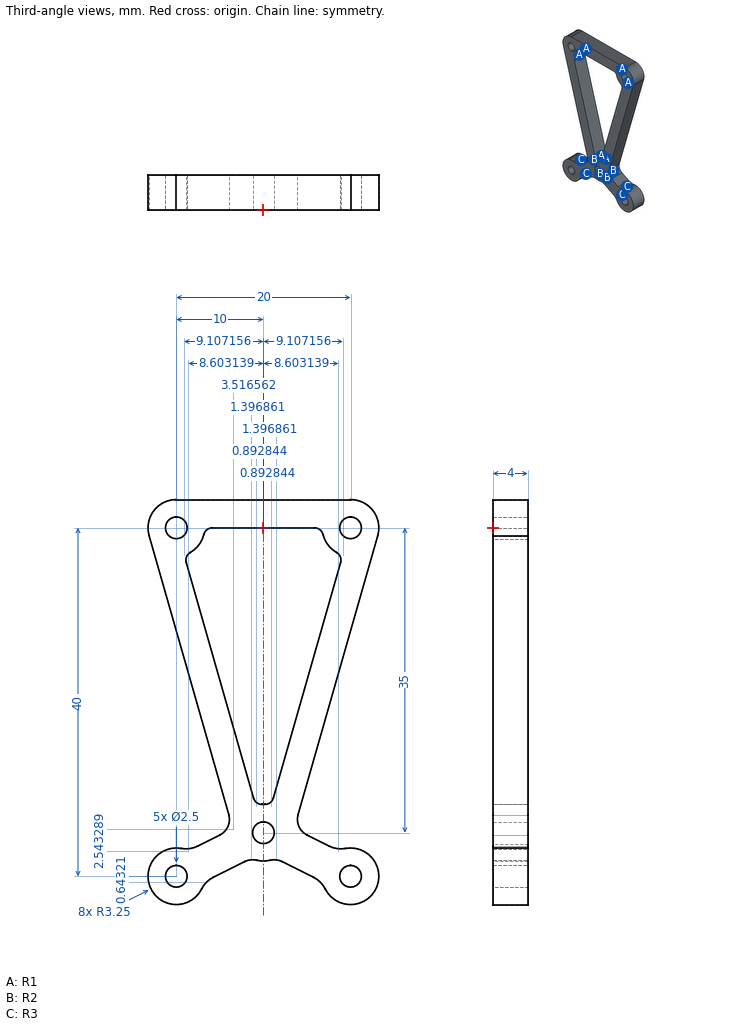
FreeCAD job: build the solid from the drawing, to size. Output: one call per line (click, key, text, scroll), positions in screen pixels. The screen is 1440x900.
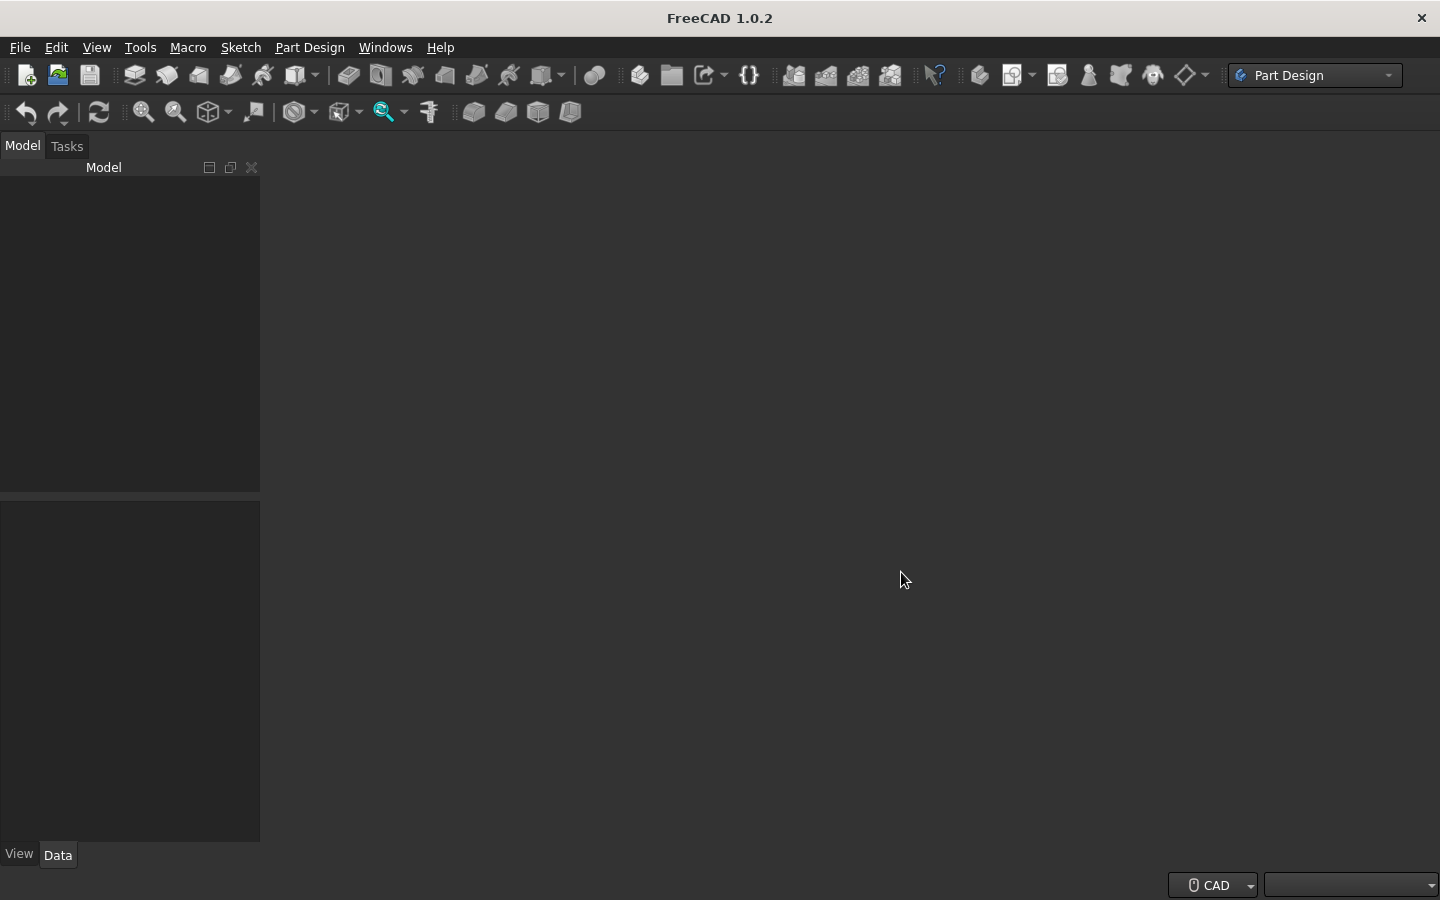
key(ctrl+n)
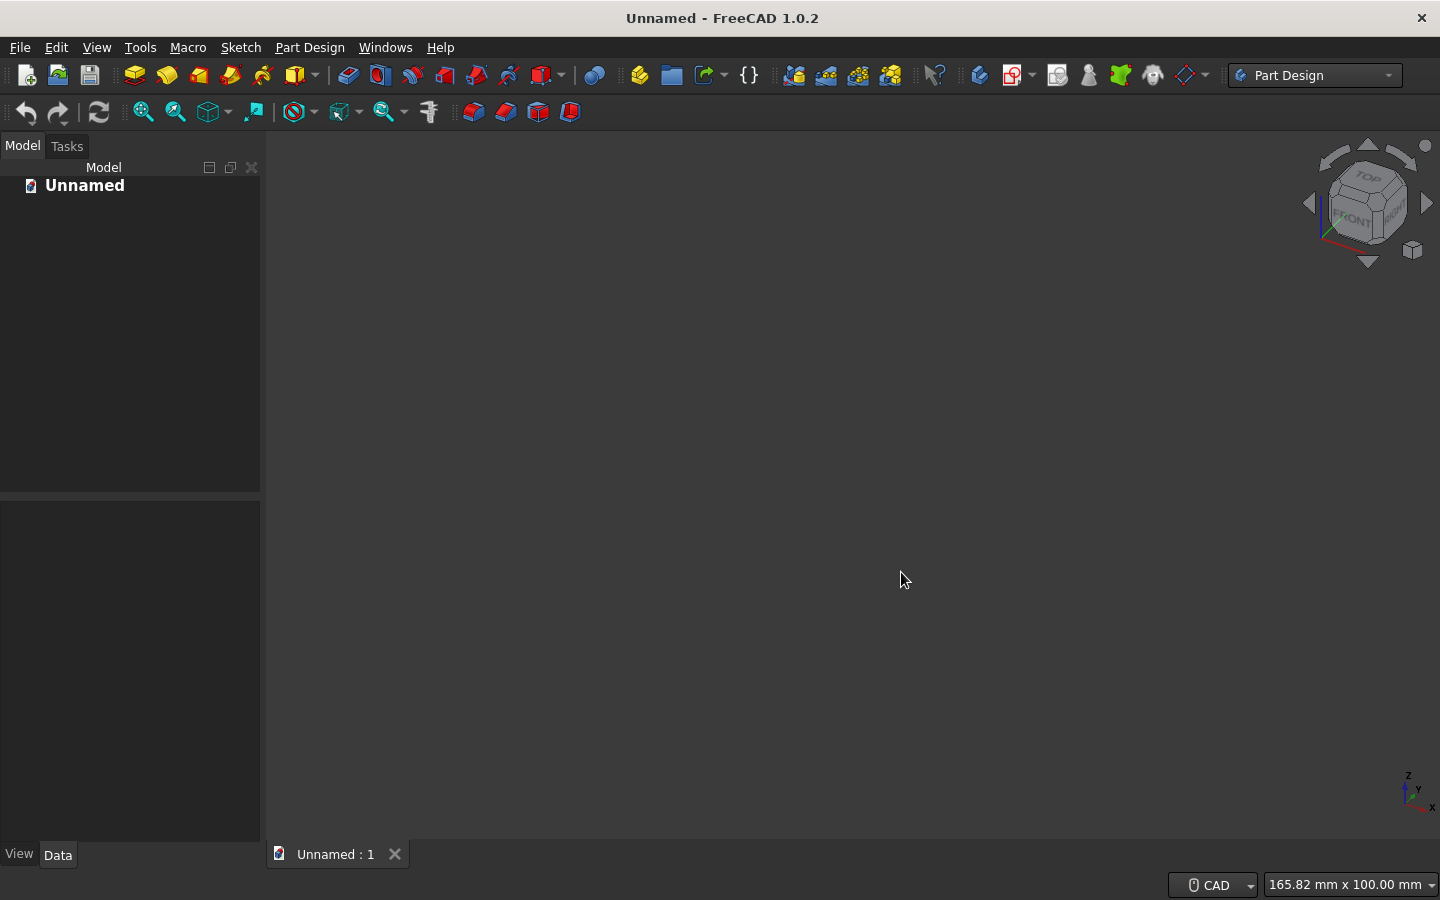
click(1012, 76)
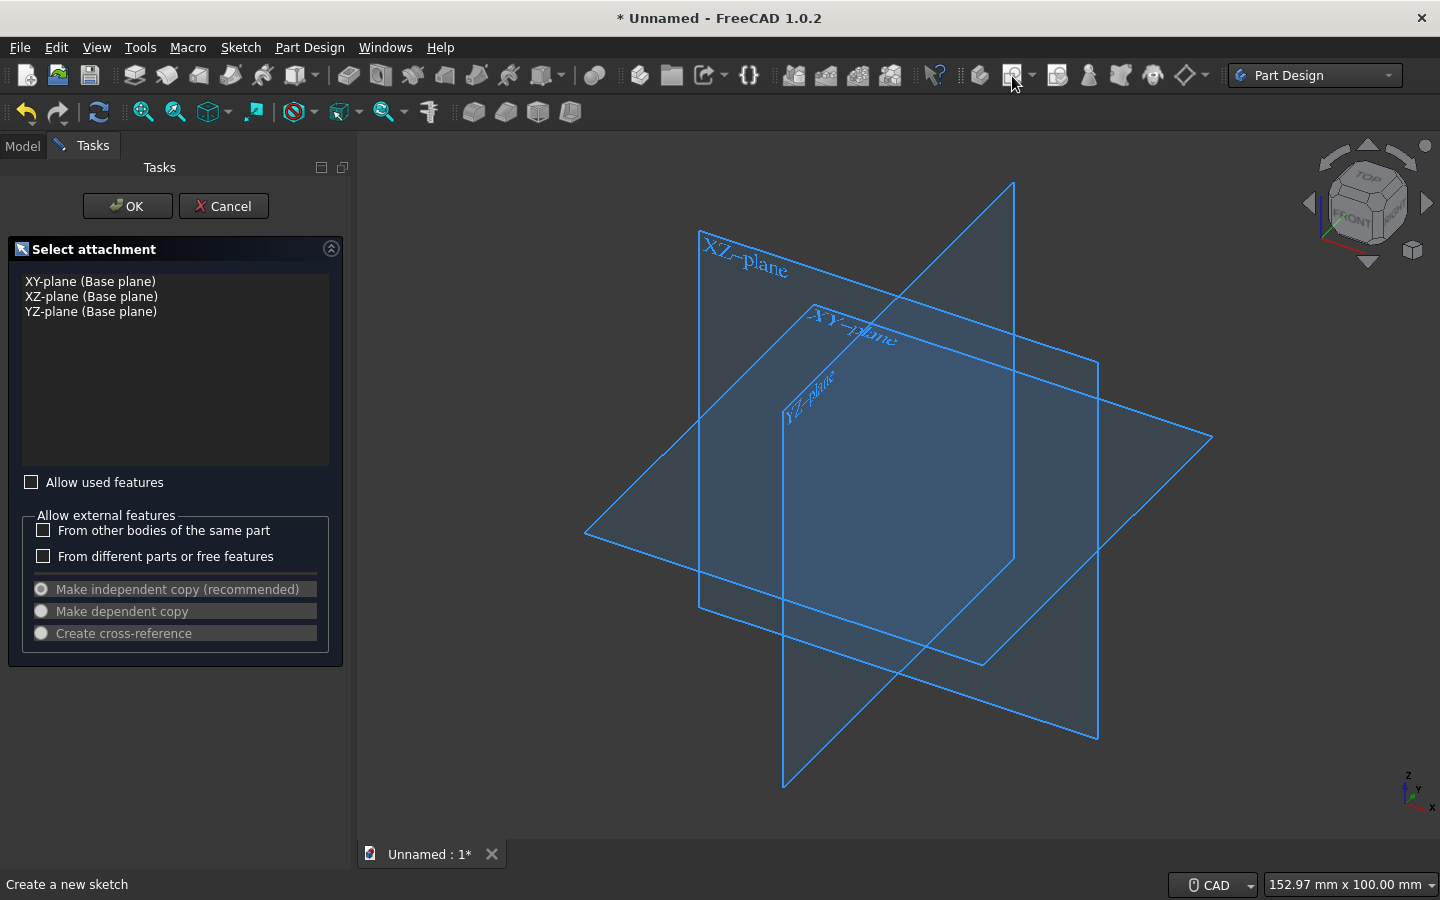
click(82, 296)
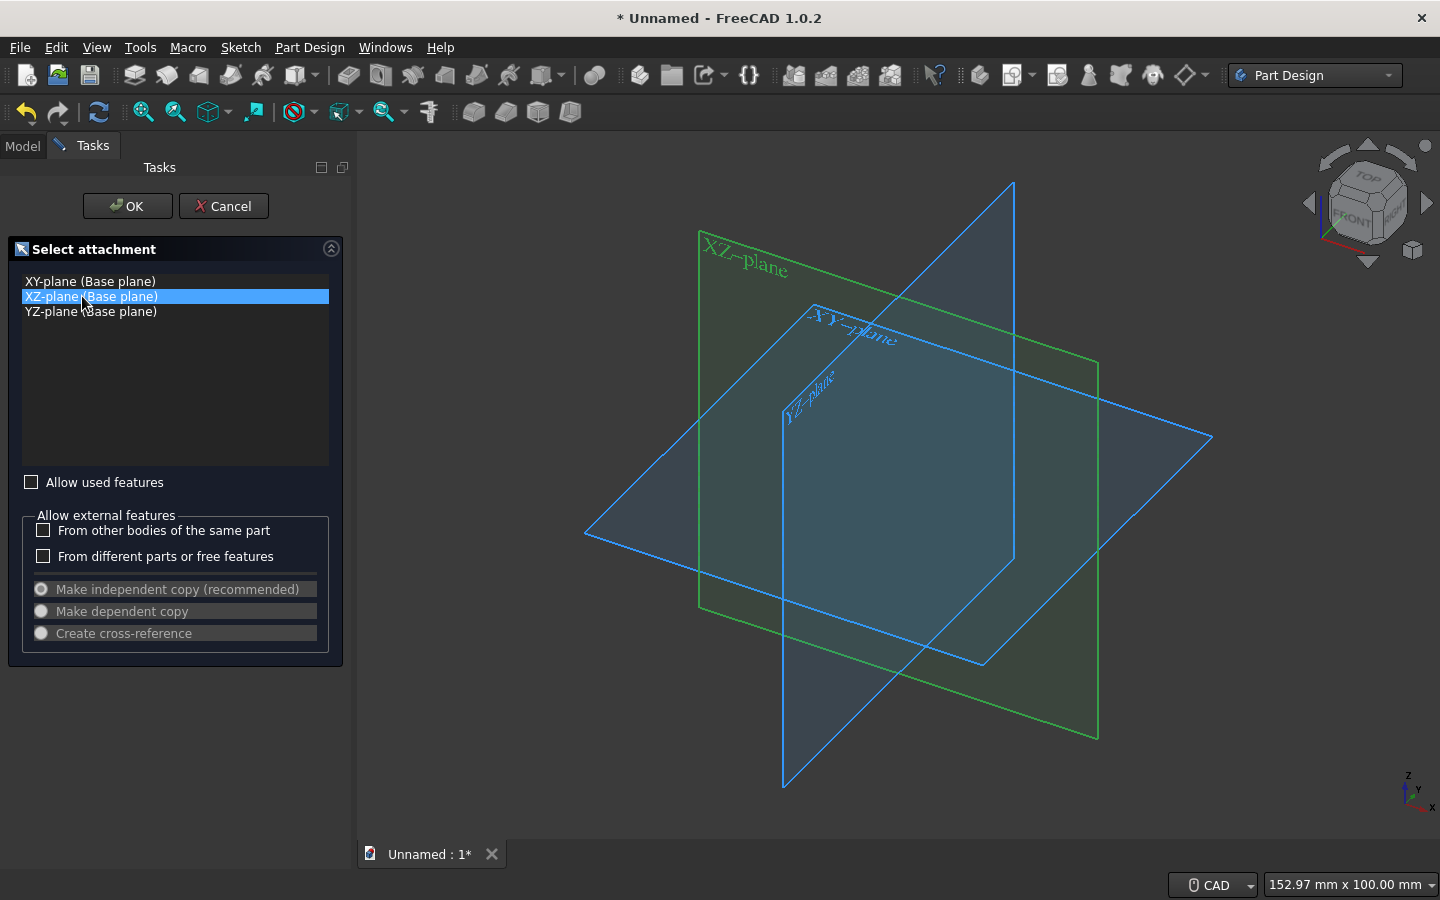
click(128, 206)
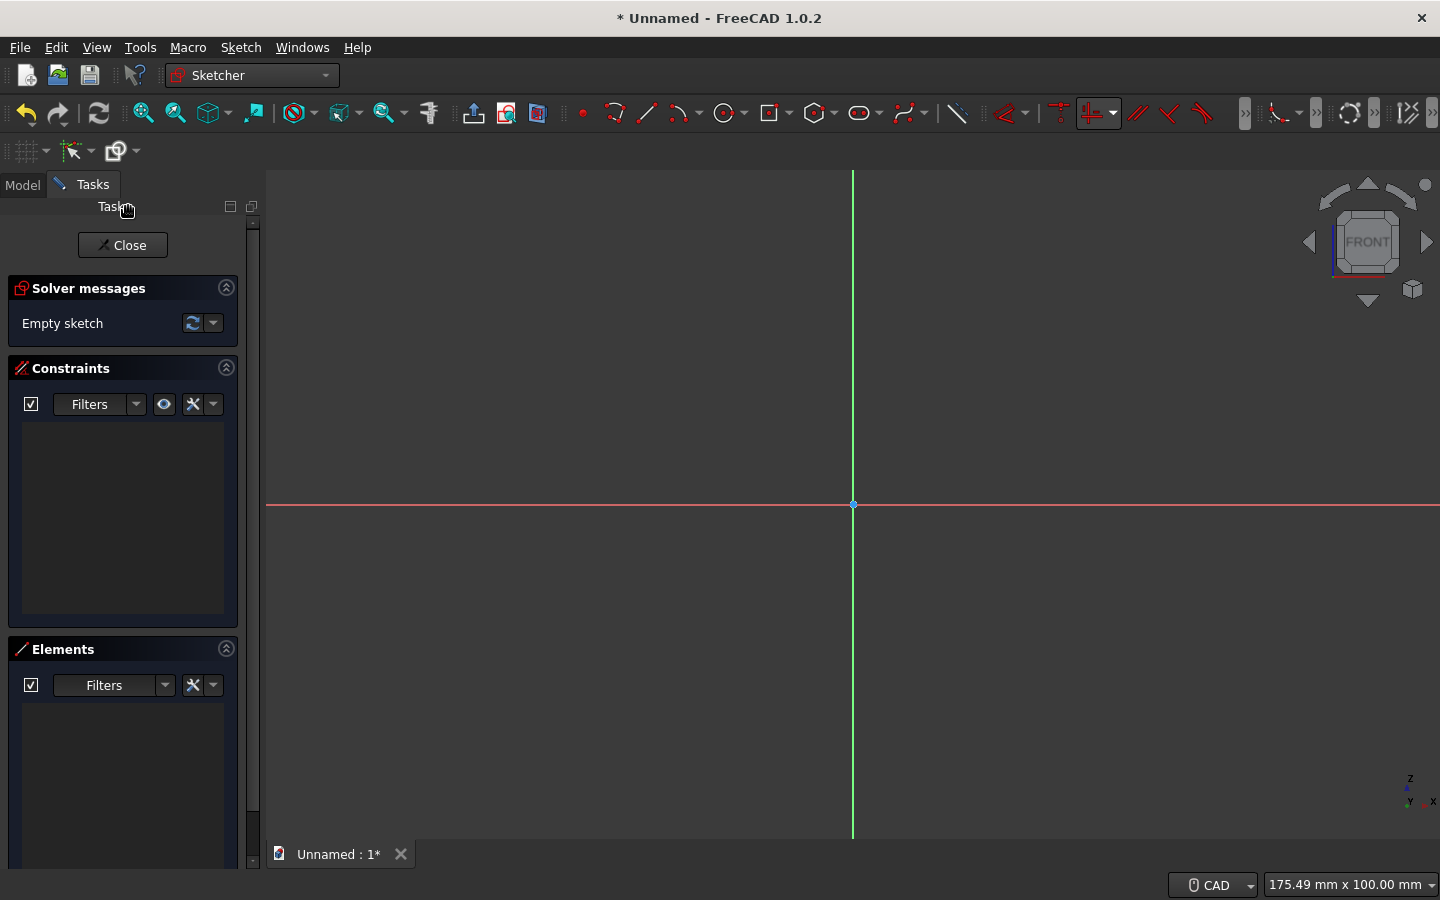
scroll(992, 811, up, 2)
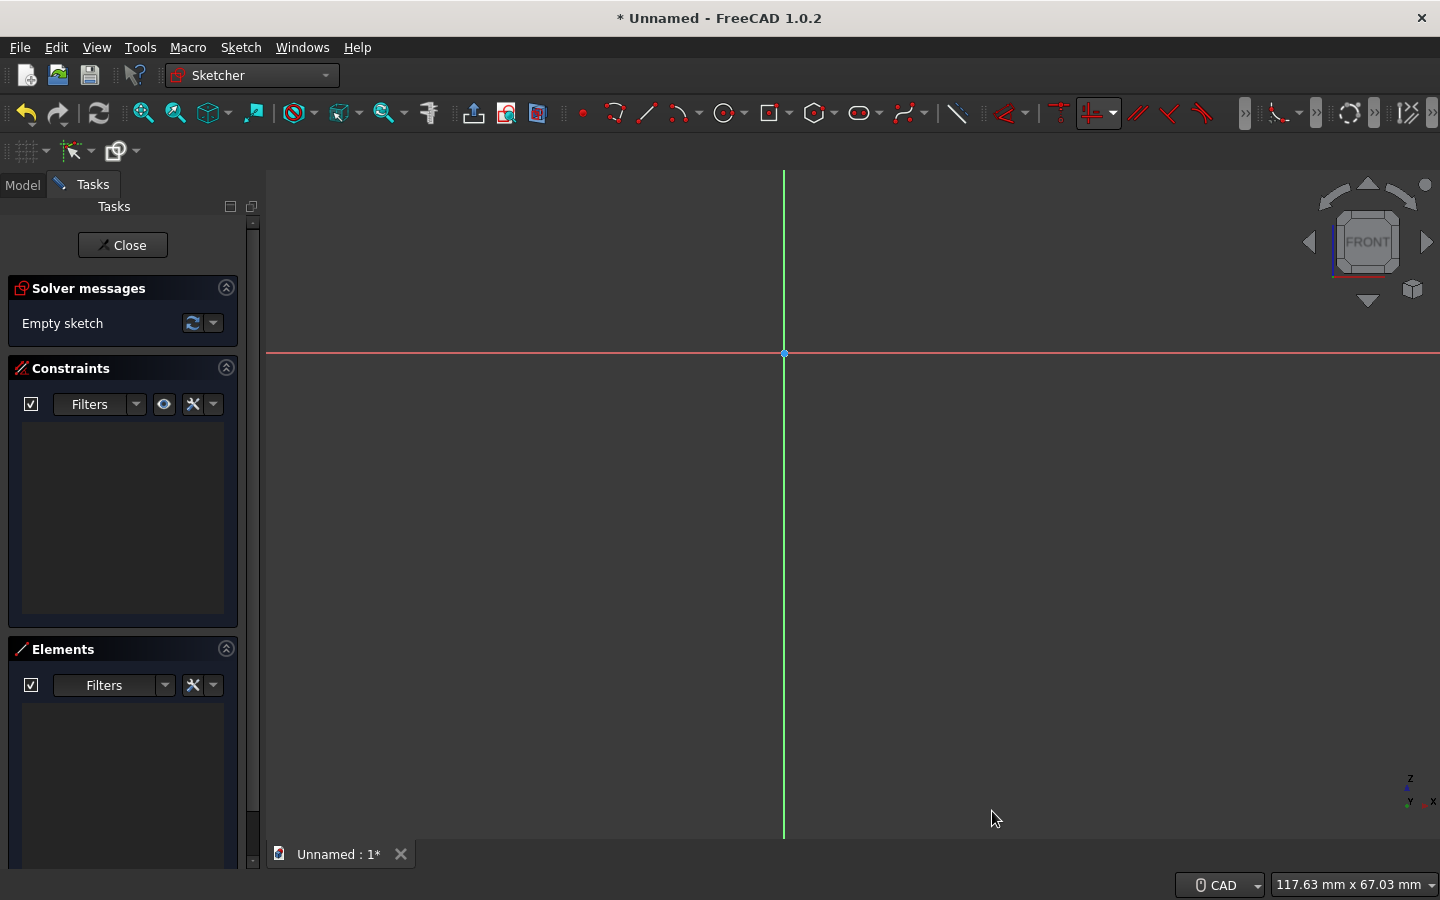
click(616, 114)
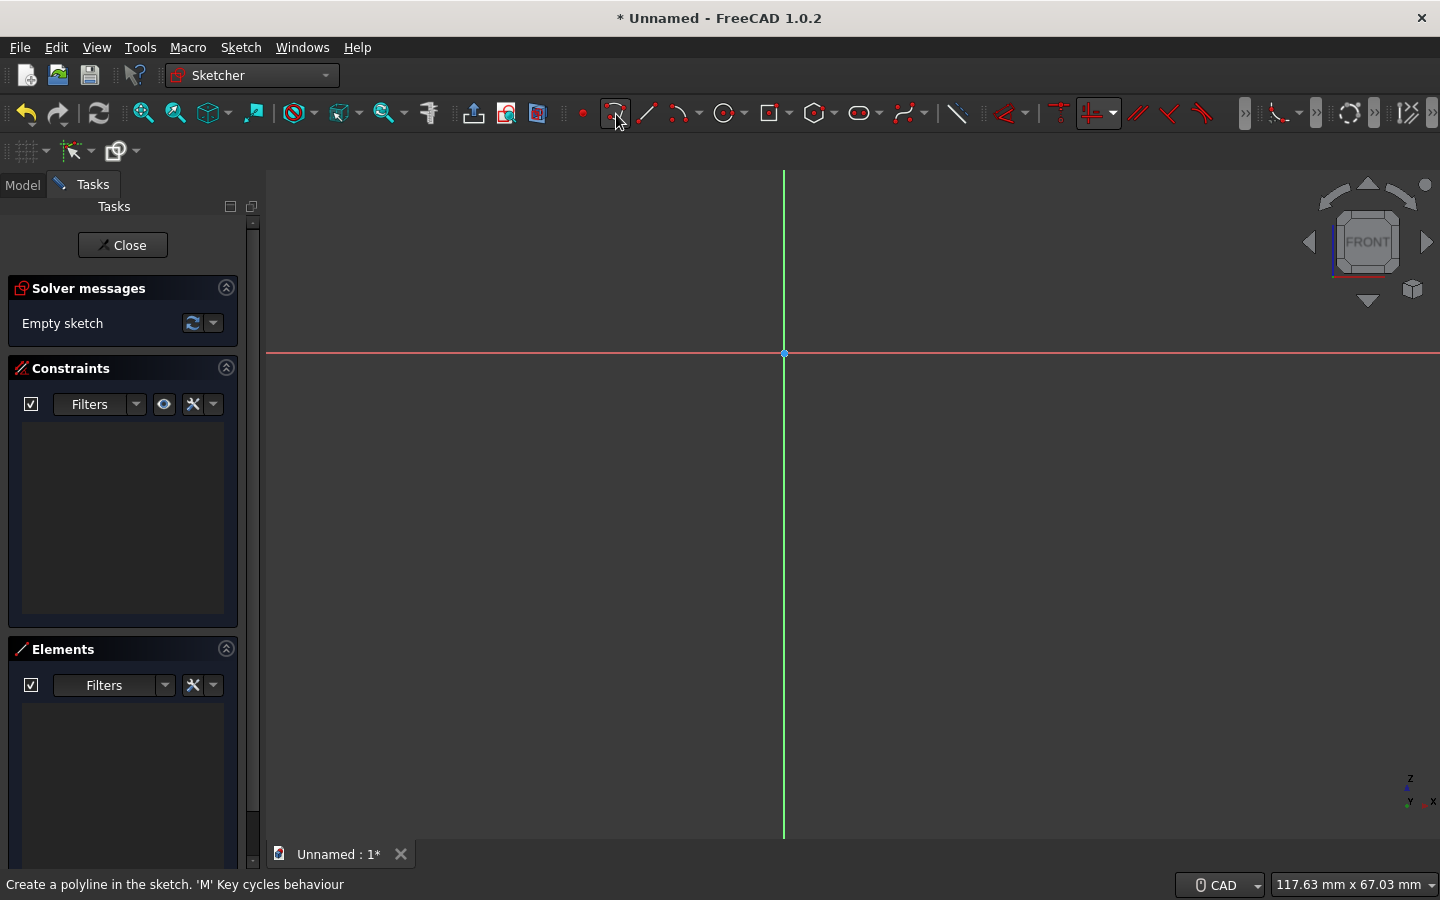
click(698, 723)
click(749, 698)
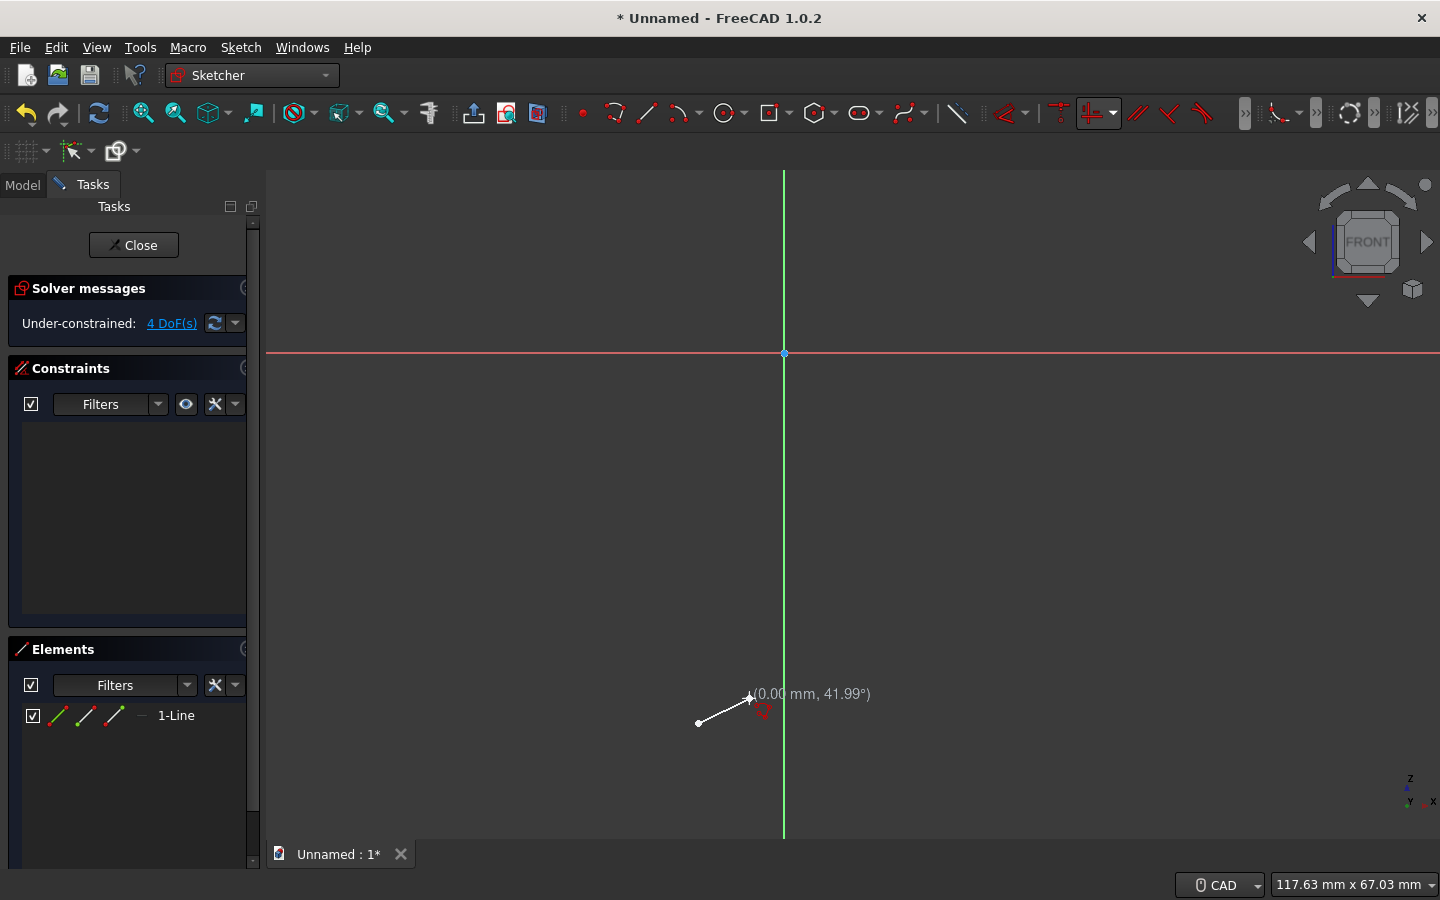
scroll(653, 362, up, 3)